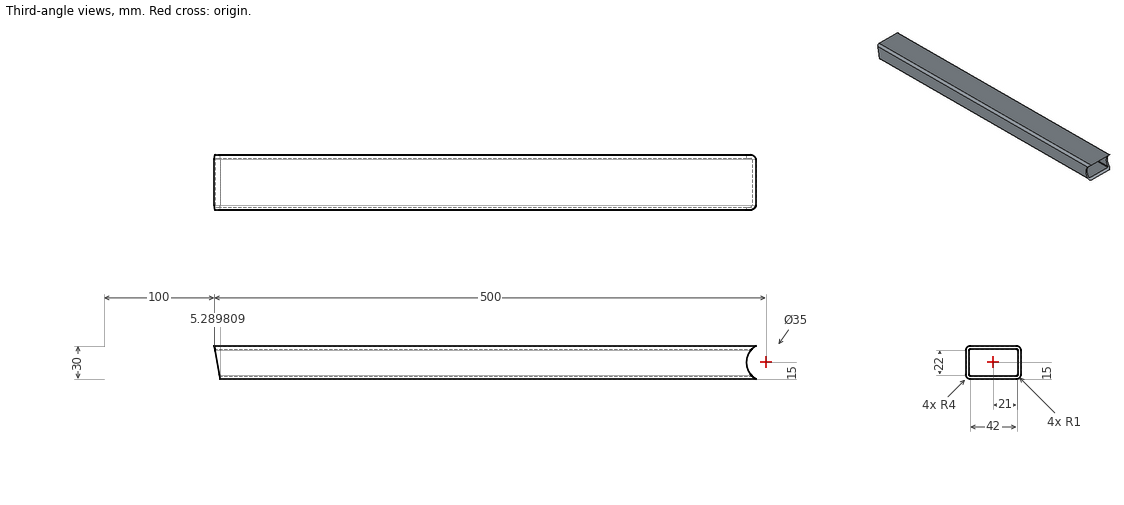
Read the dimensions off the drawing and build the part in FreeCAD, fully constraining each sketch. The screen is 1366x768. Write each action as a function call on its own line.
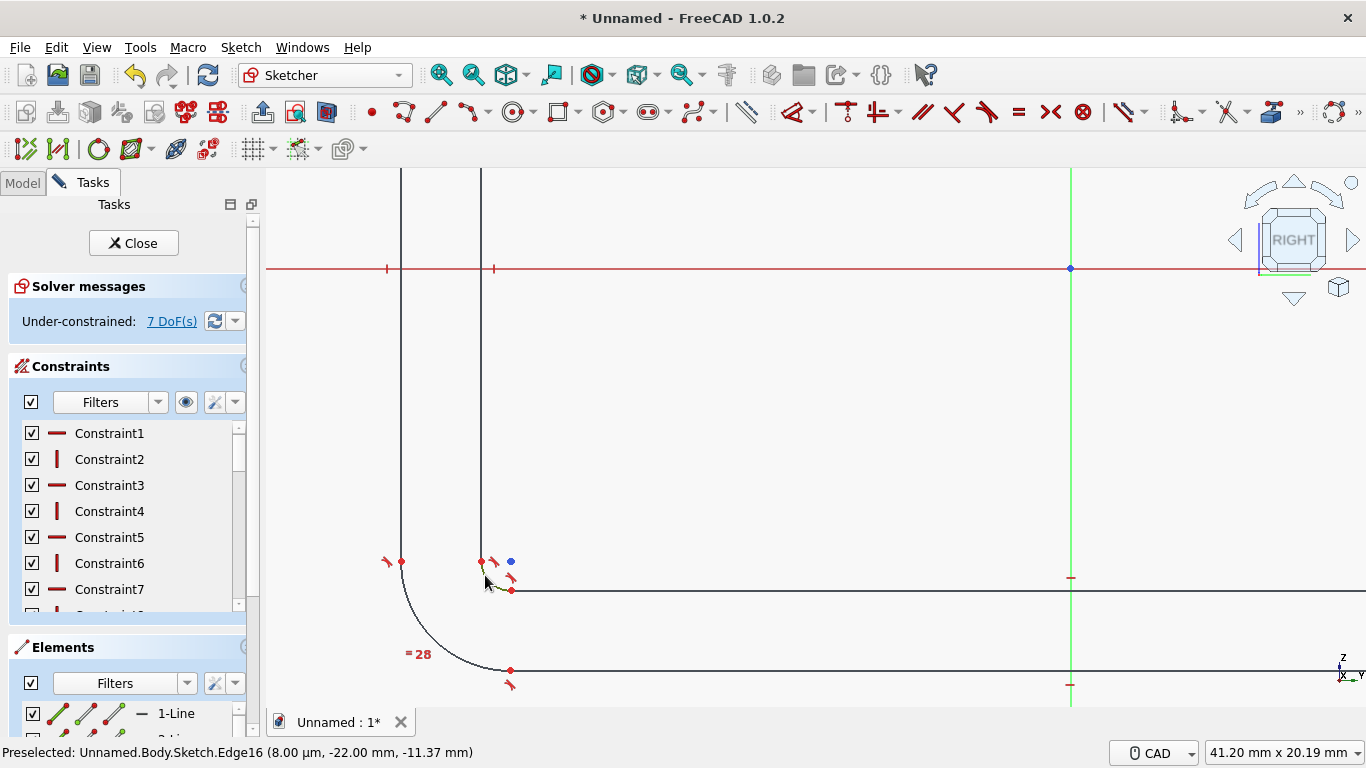
click(1020, 112)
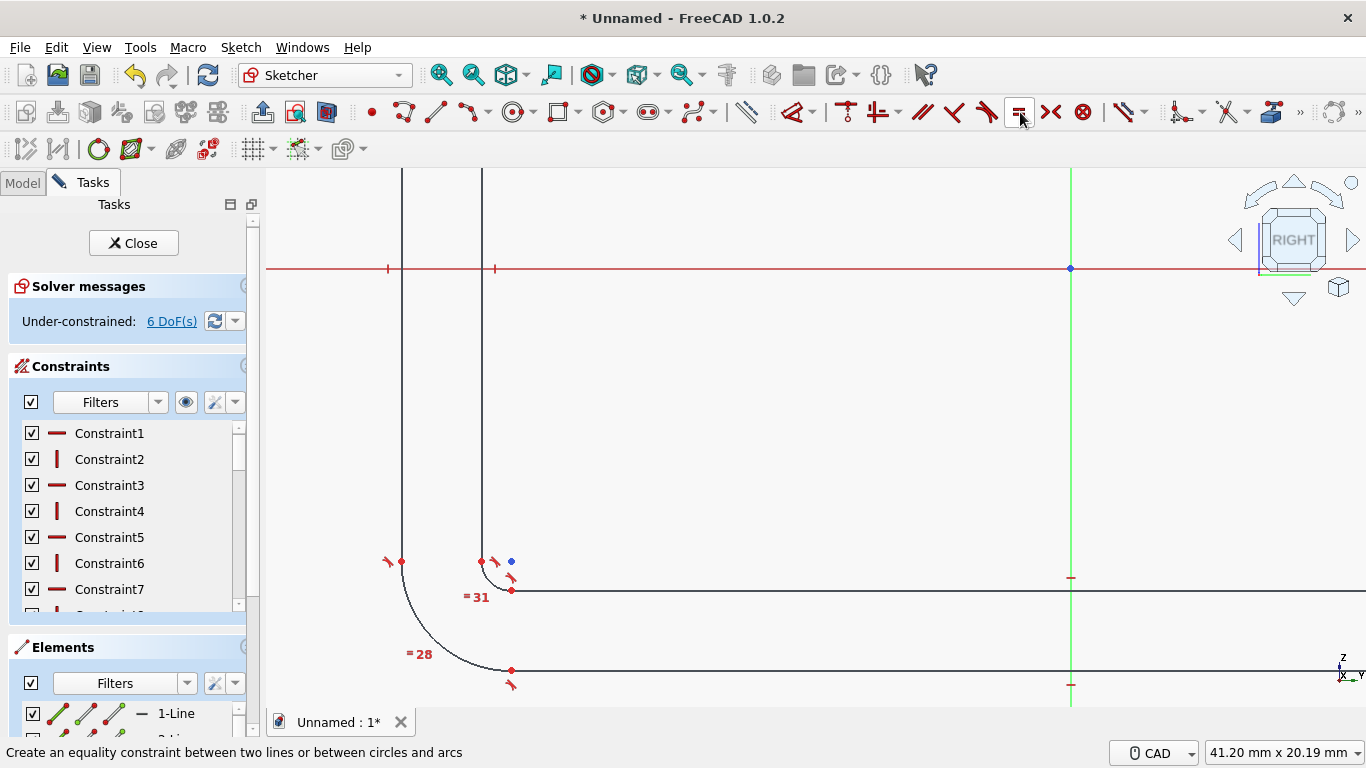
key(d)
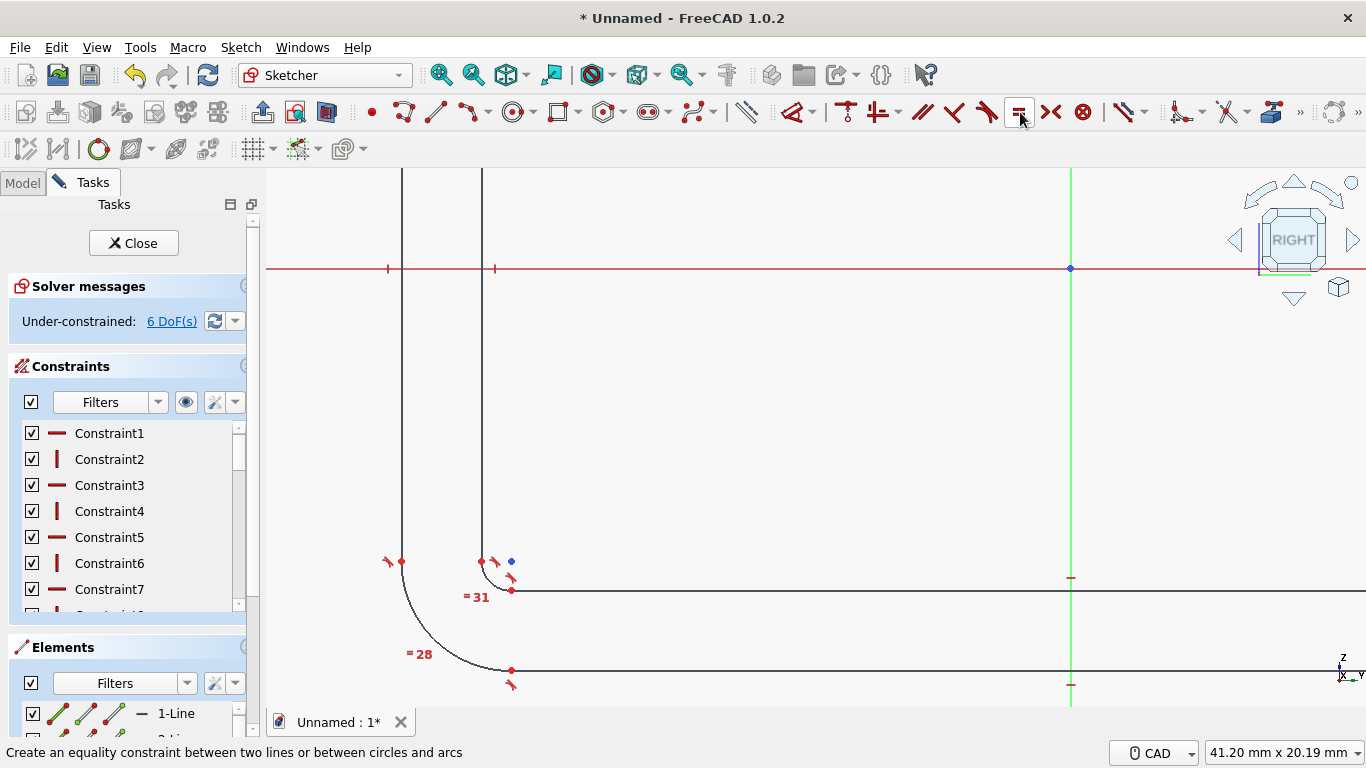
click(413, 611)
click(384, 625)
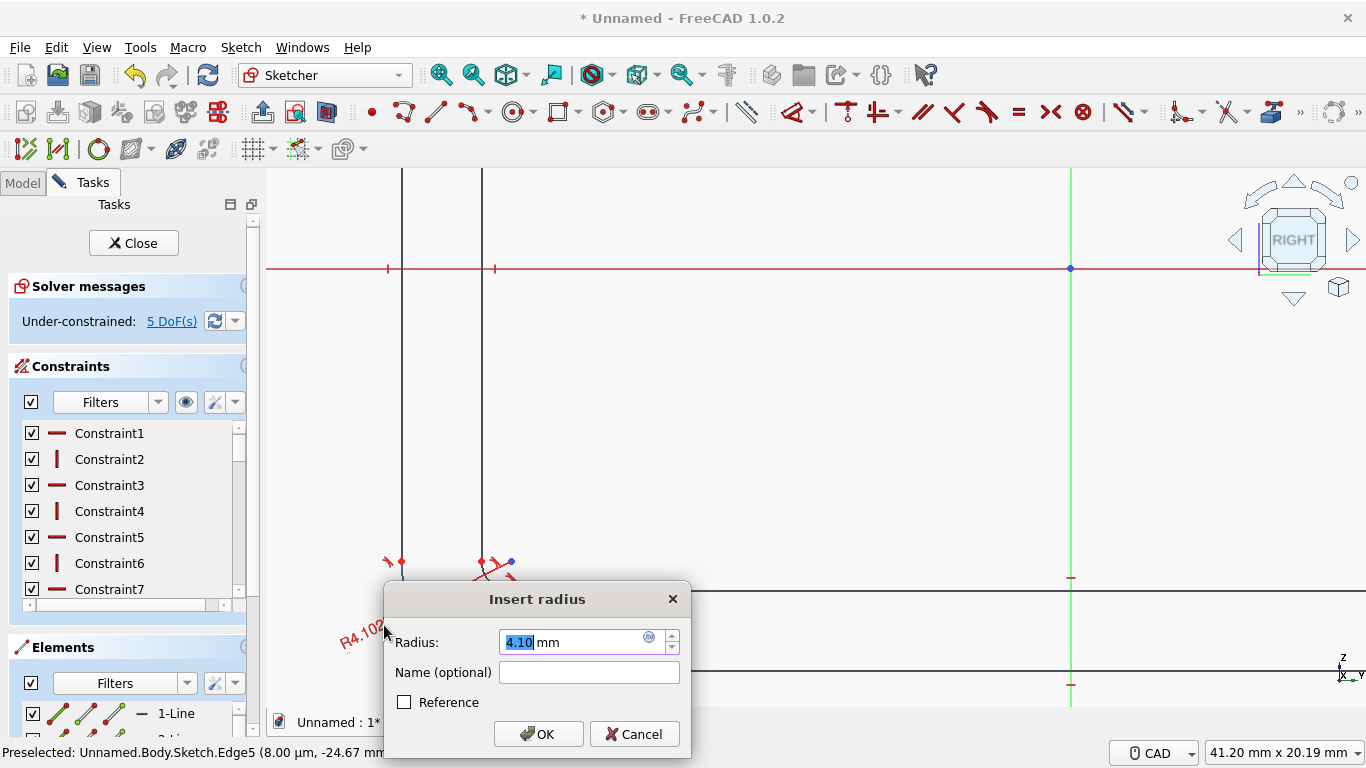
text(4)
key(Return)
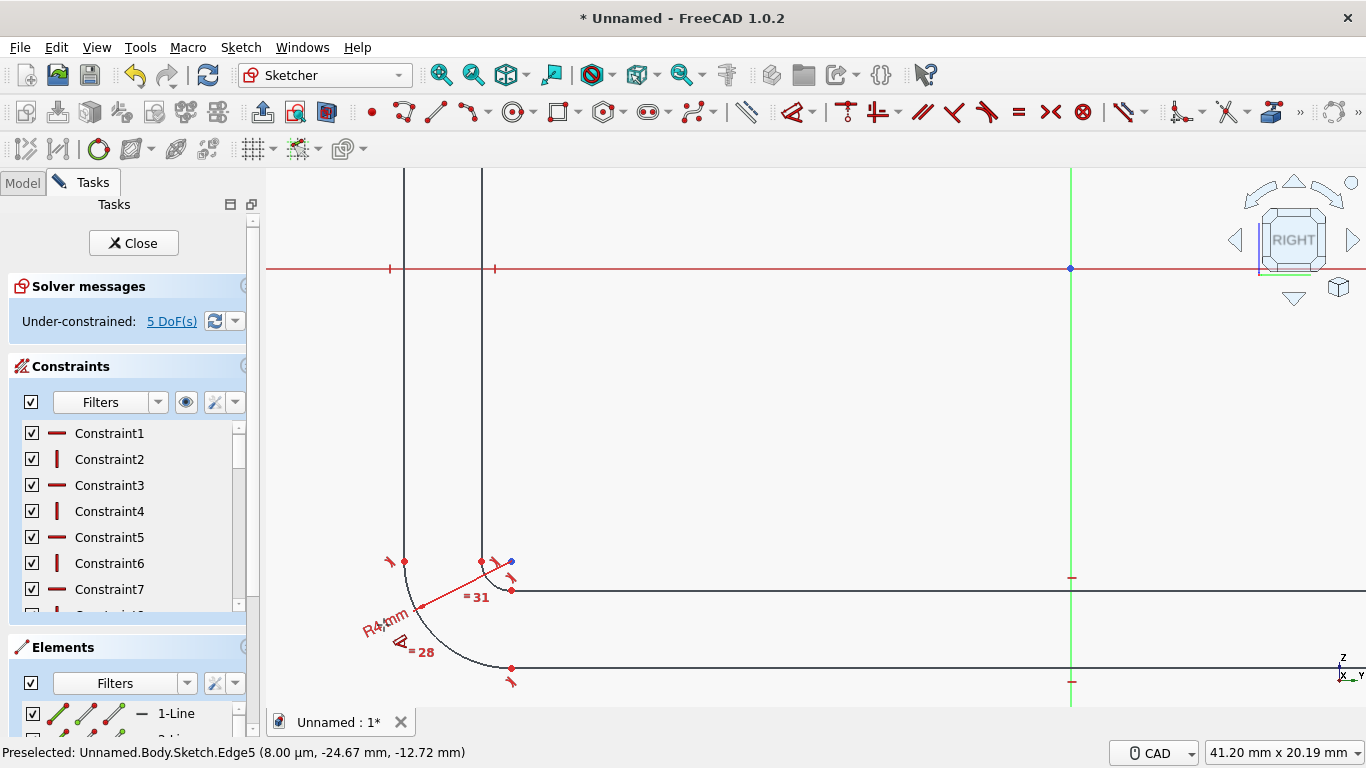
scroll(484, 575, down, 4)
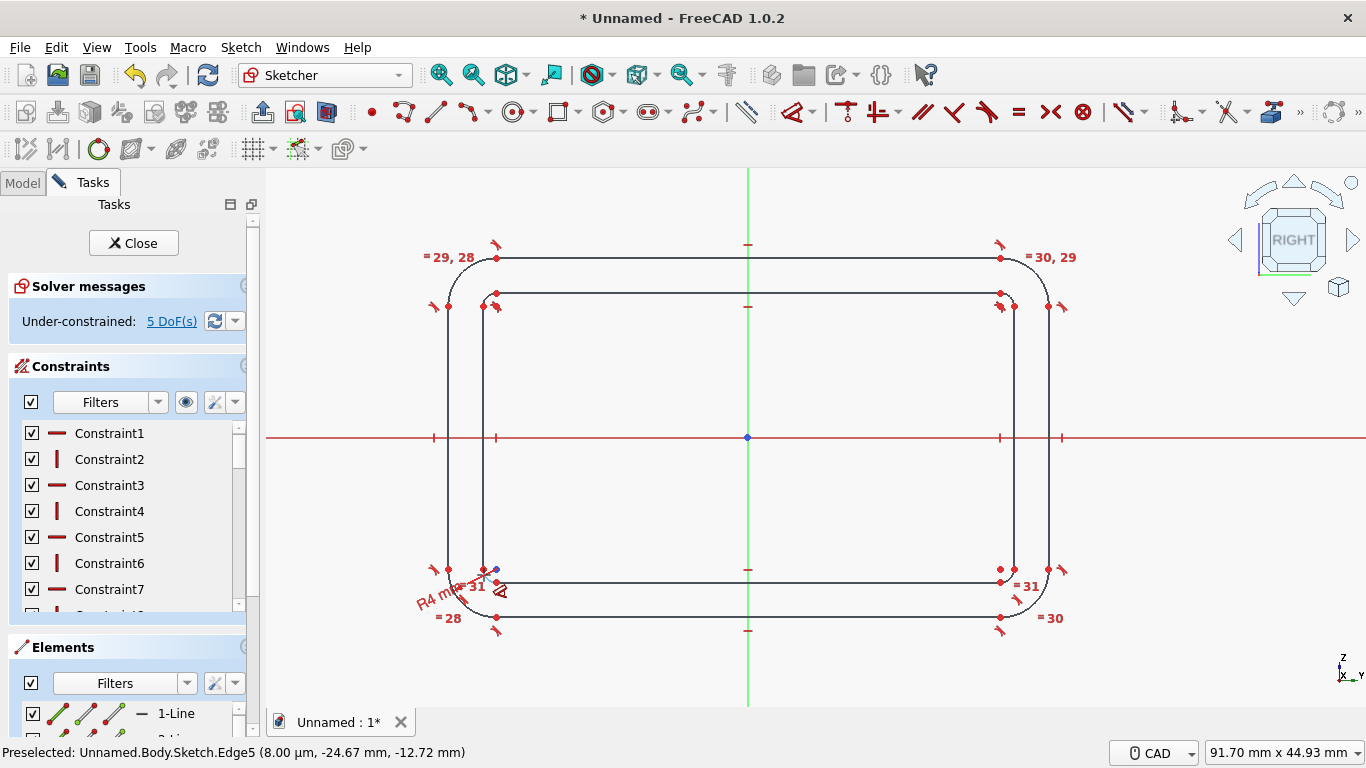
scroll(1007, 581, up, 6)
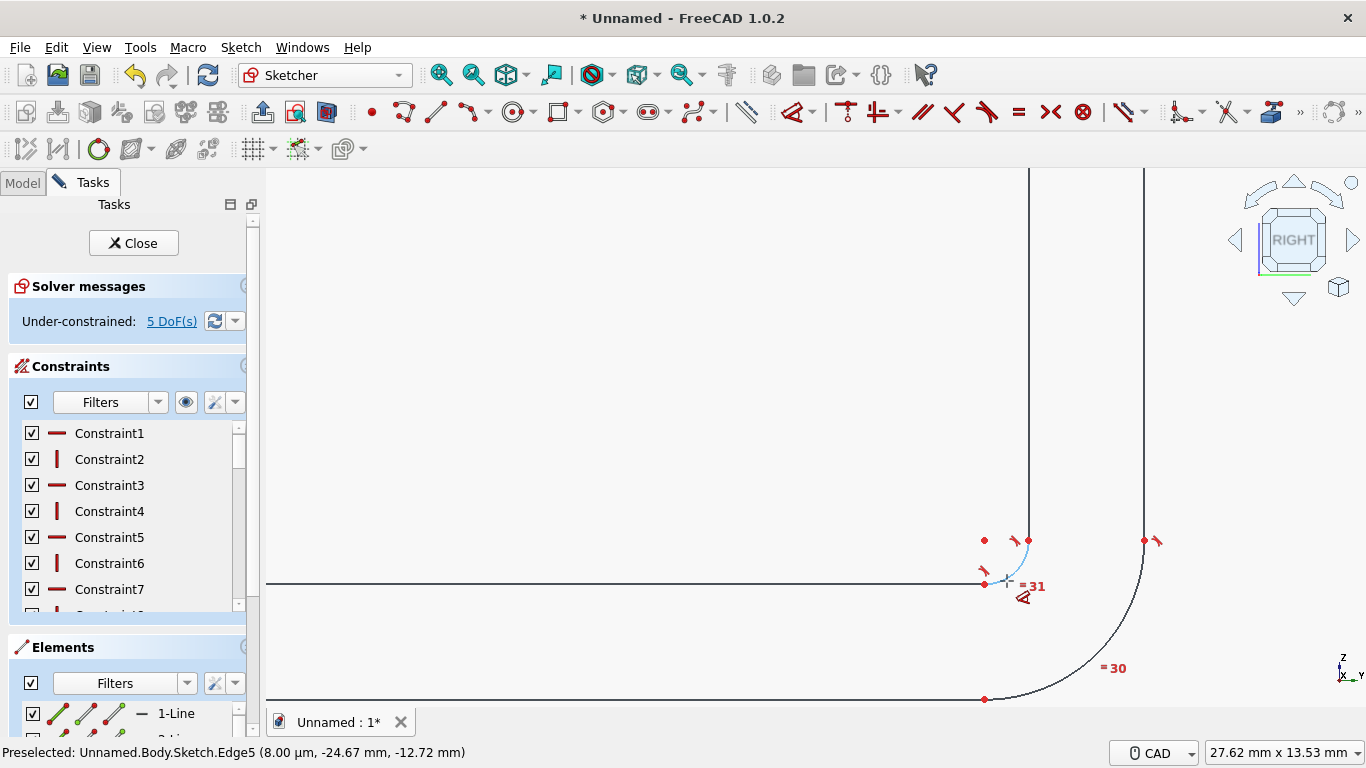
click(1005, 580)
click(1019, 609)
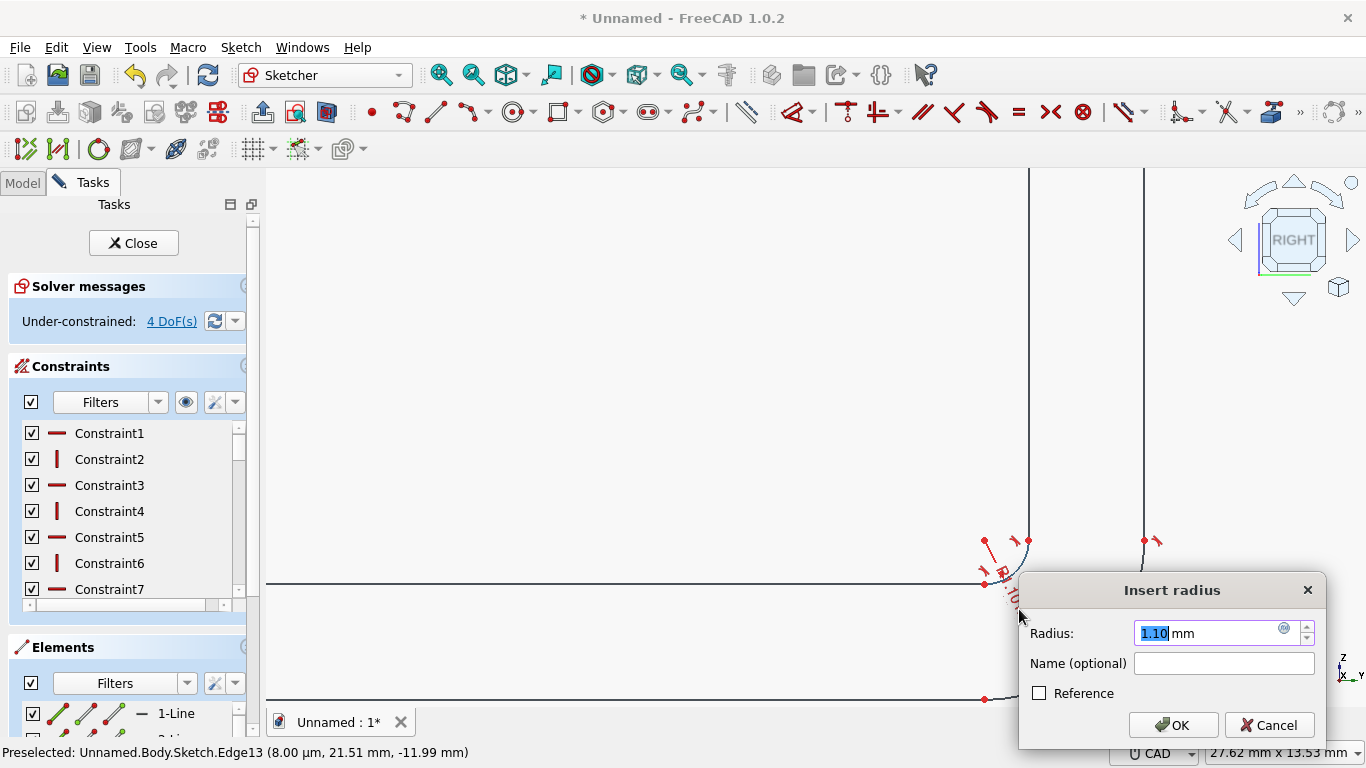
text(1)
key(Return)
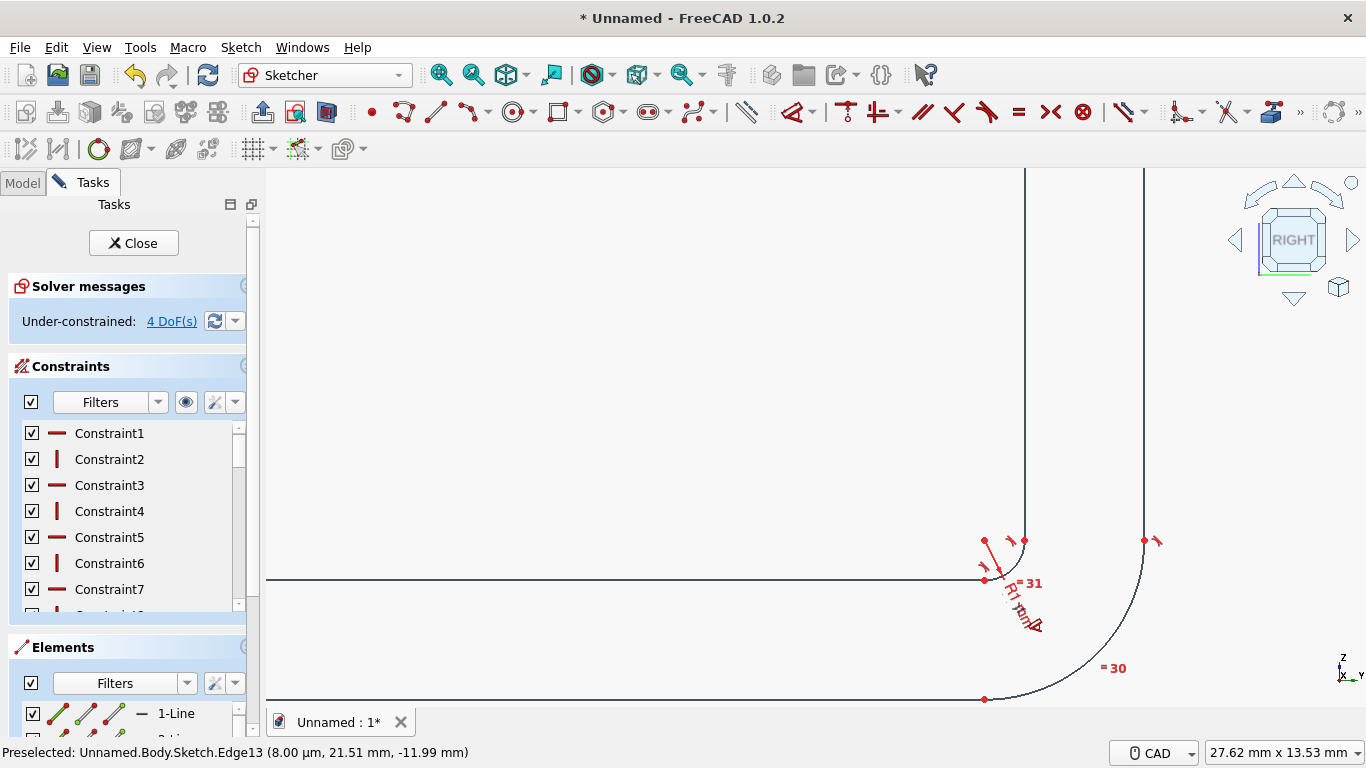
scroll(1007, 581, down, 6)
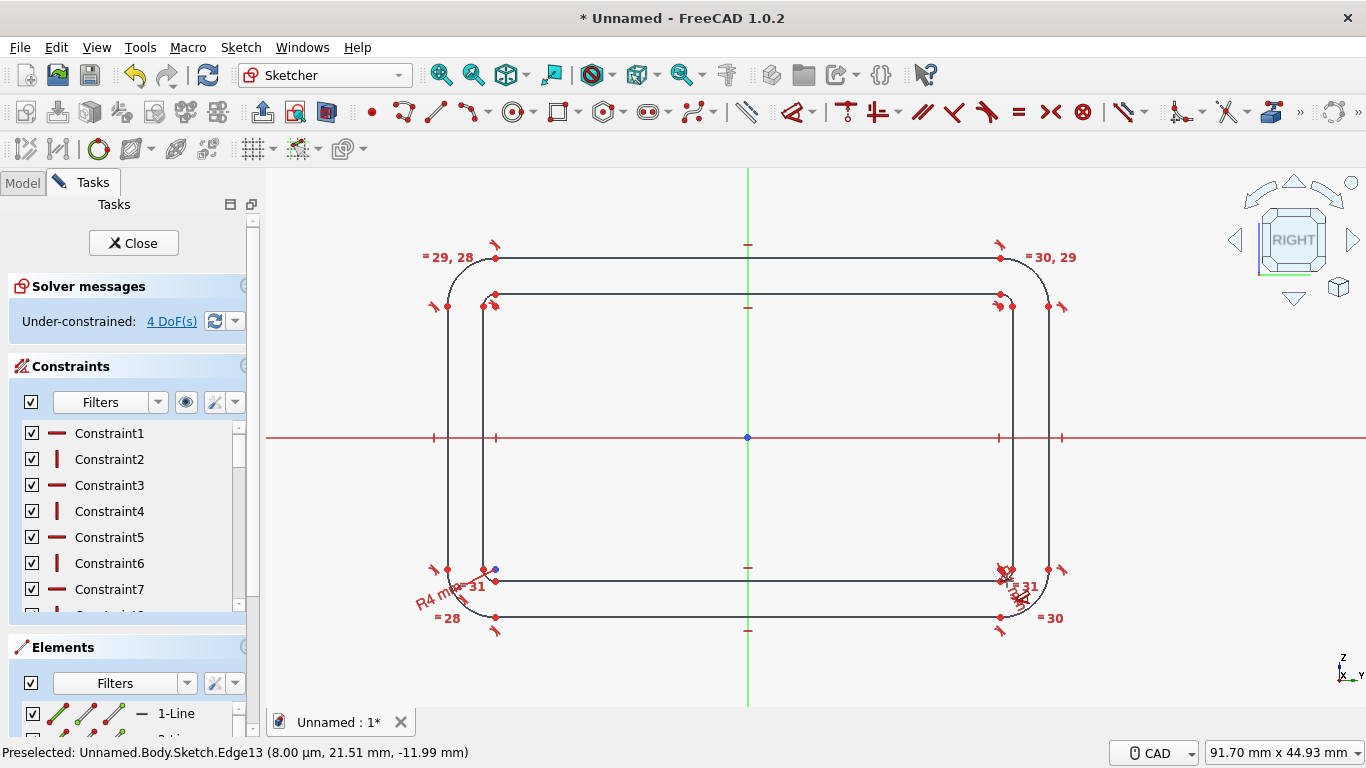
click(849, 617)
click(632, 651)